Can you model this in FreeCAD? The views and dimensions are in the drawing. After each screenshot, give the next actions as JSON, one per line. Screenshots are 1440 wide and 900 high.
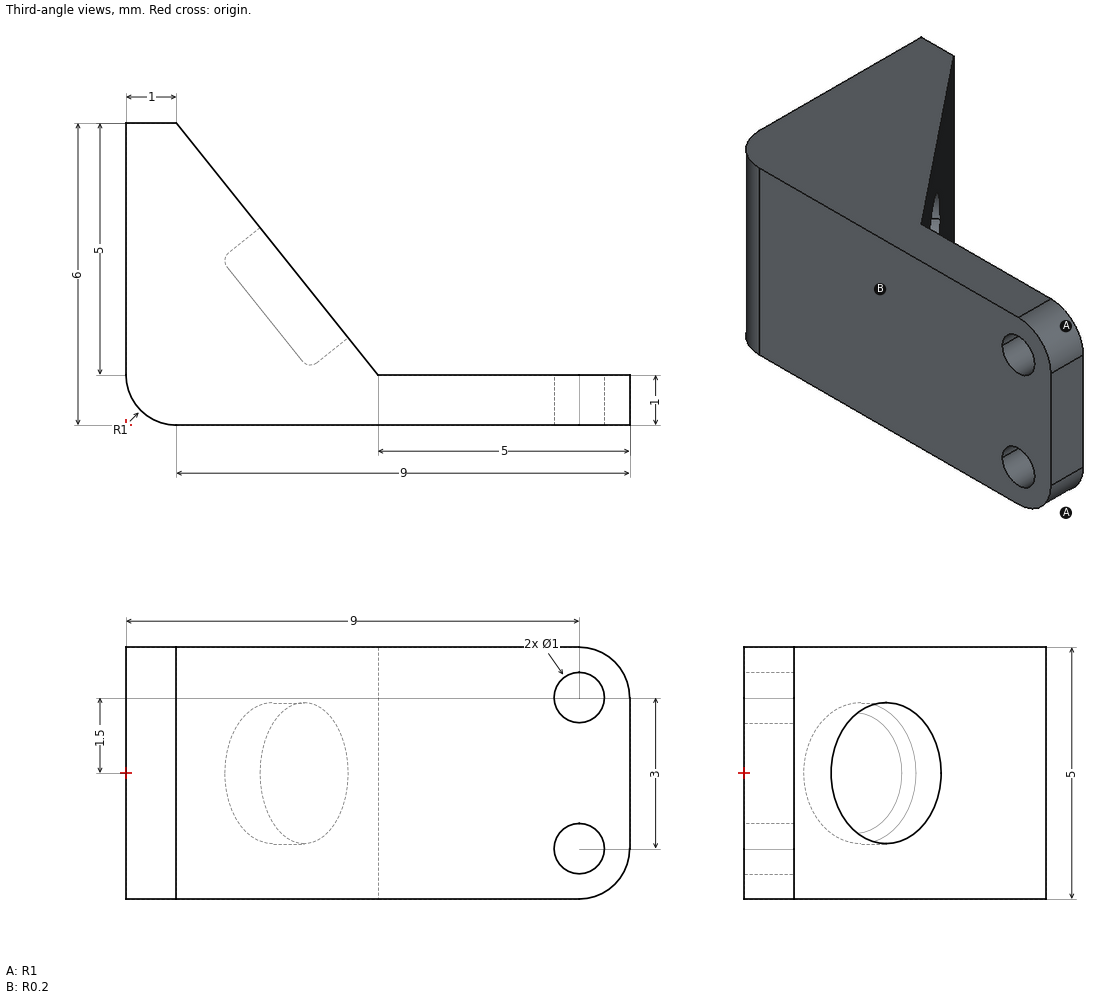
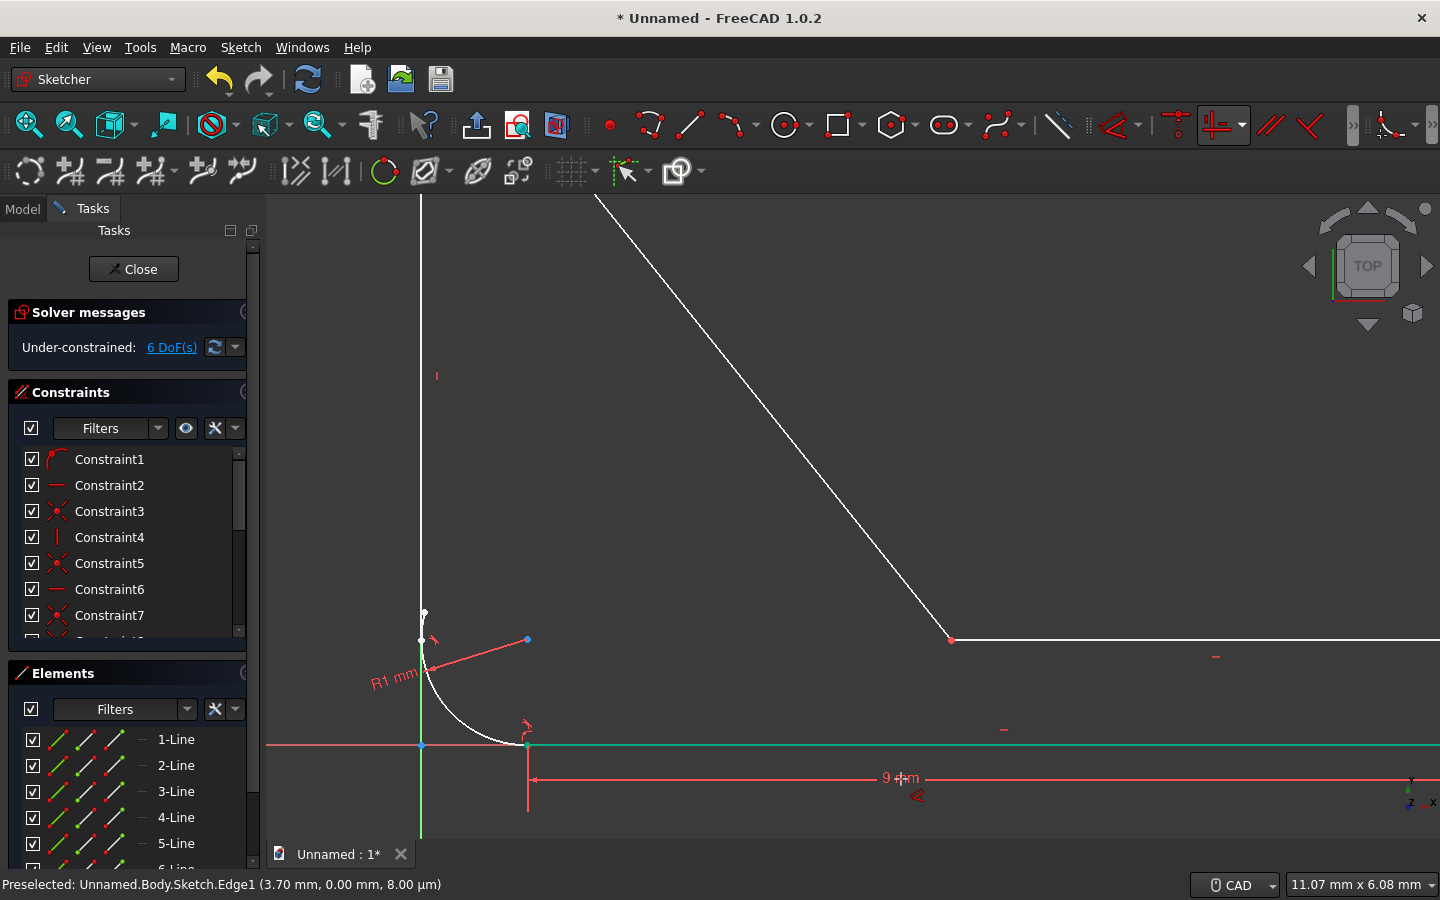
{"action": "scroll", "coordinate": [444, 698], "scroll_direction": "down", "scroll_amount": 2}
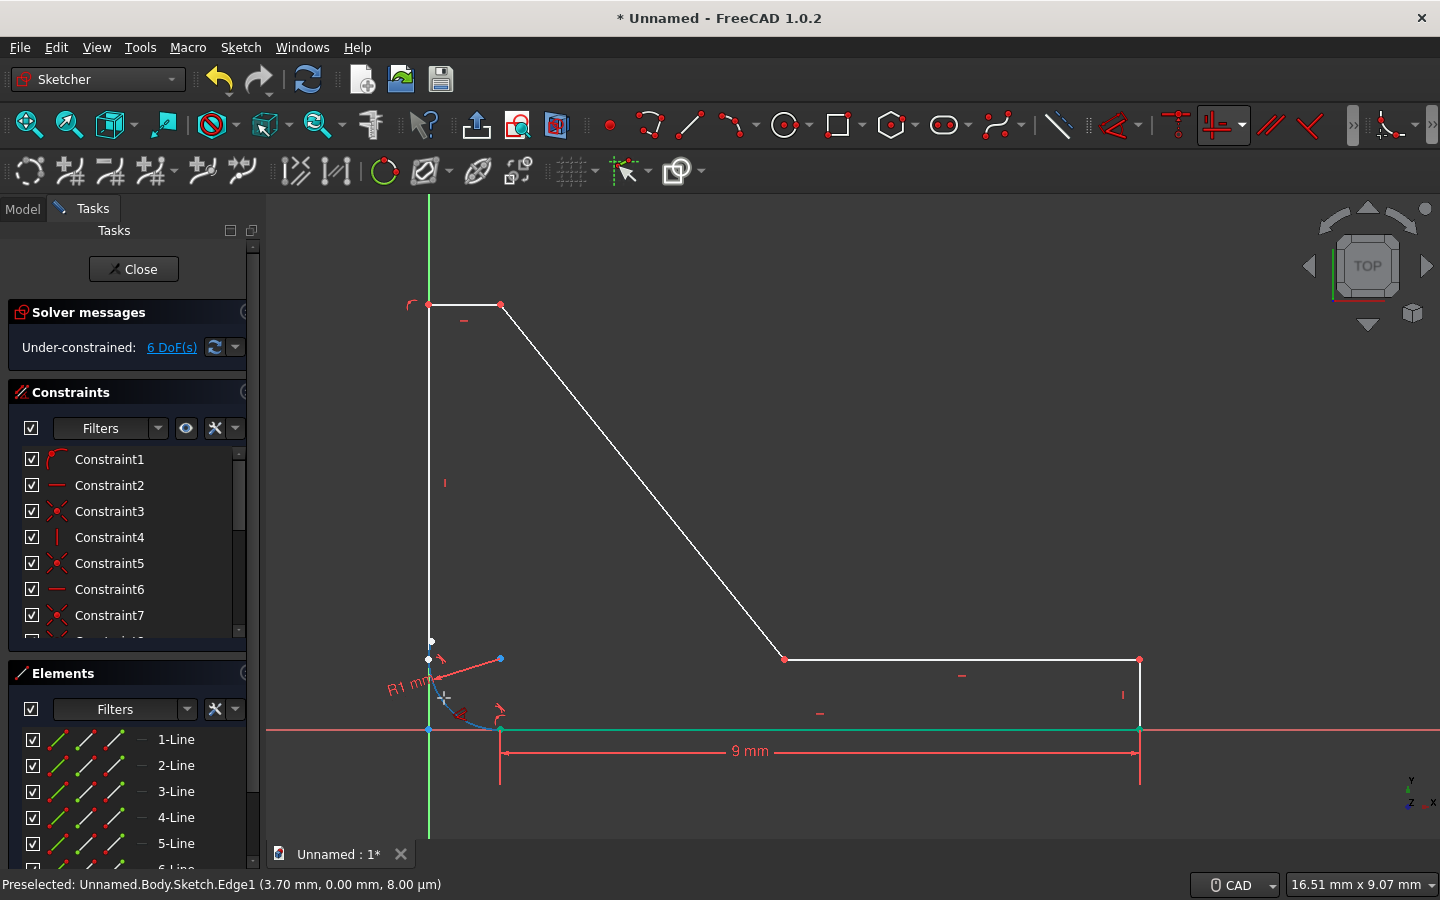
{"action": "left_click", "coordinate": [1140, 709]}
{"action": "left_click", "coordinate": [1174, 695]}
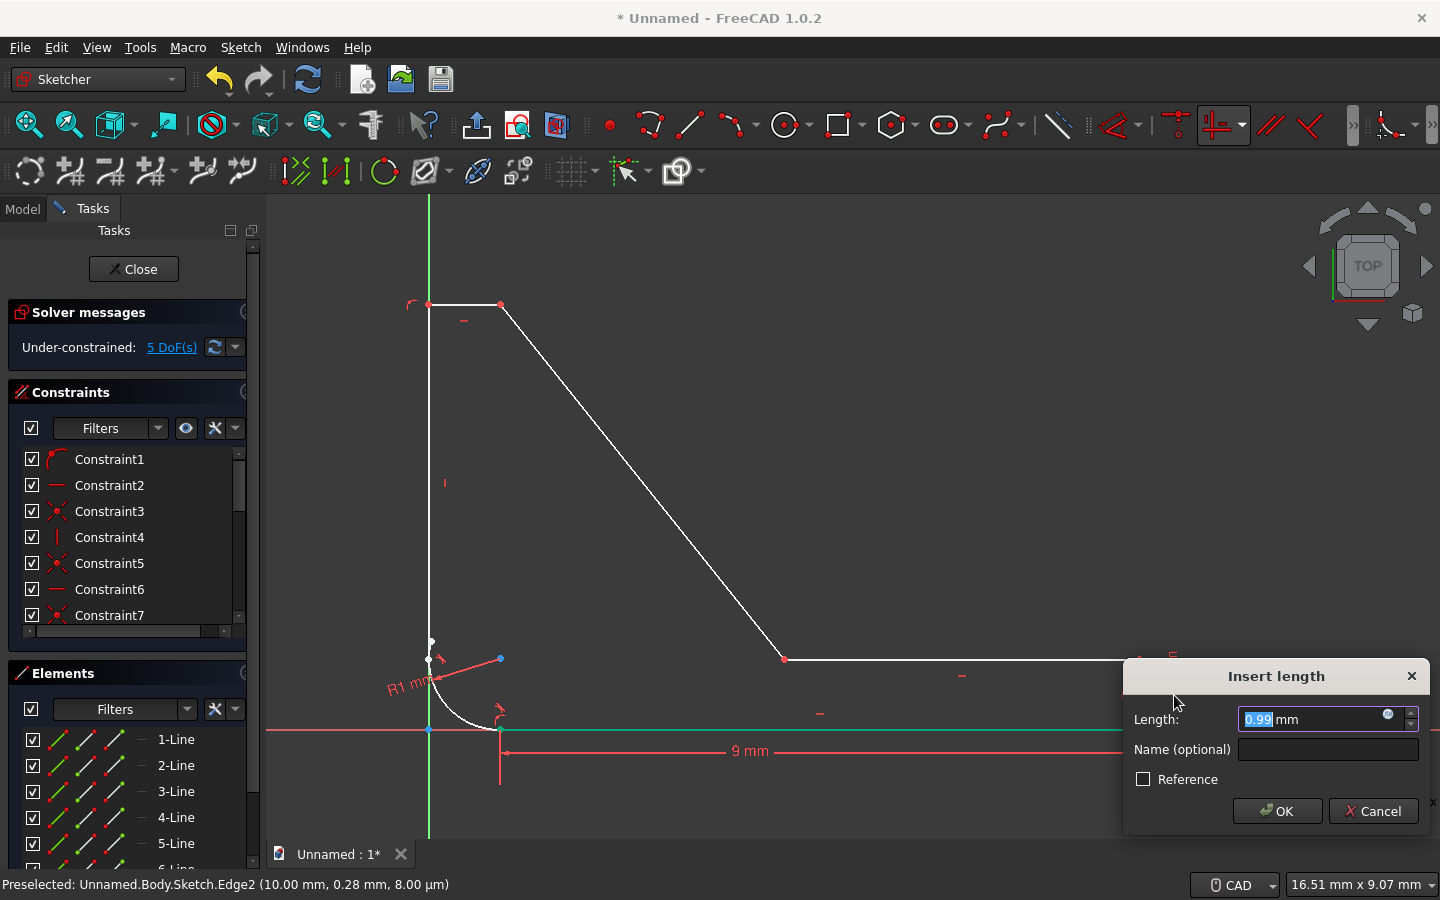
{"action": "type", "text": "1"}
{"action": "key", "text": "Return"}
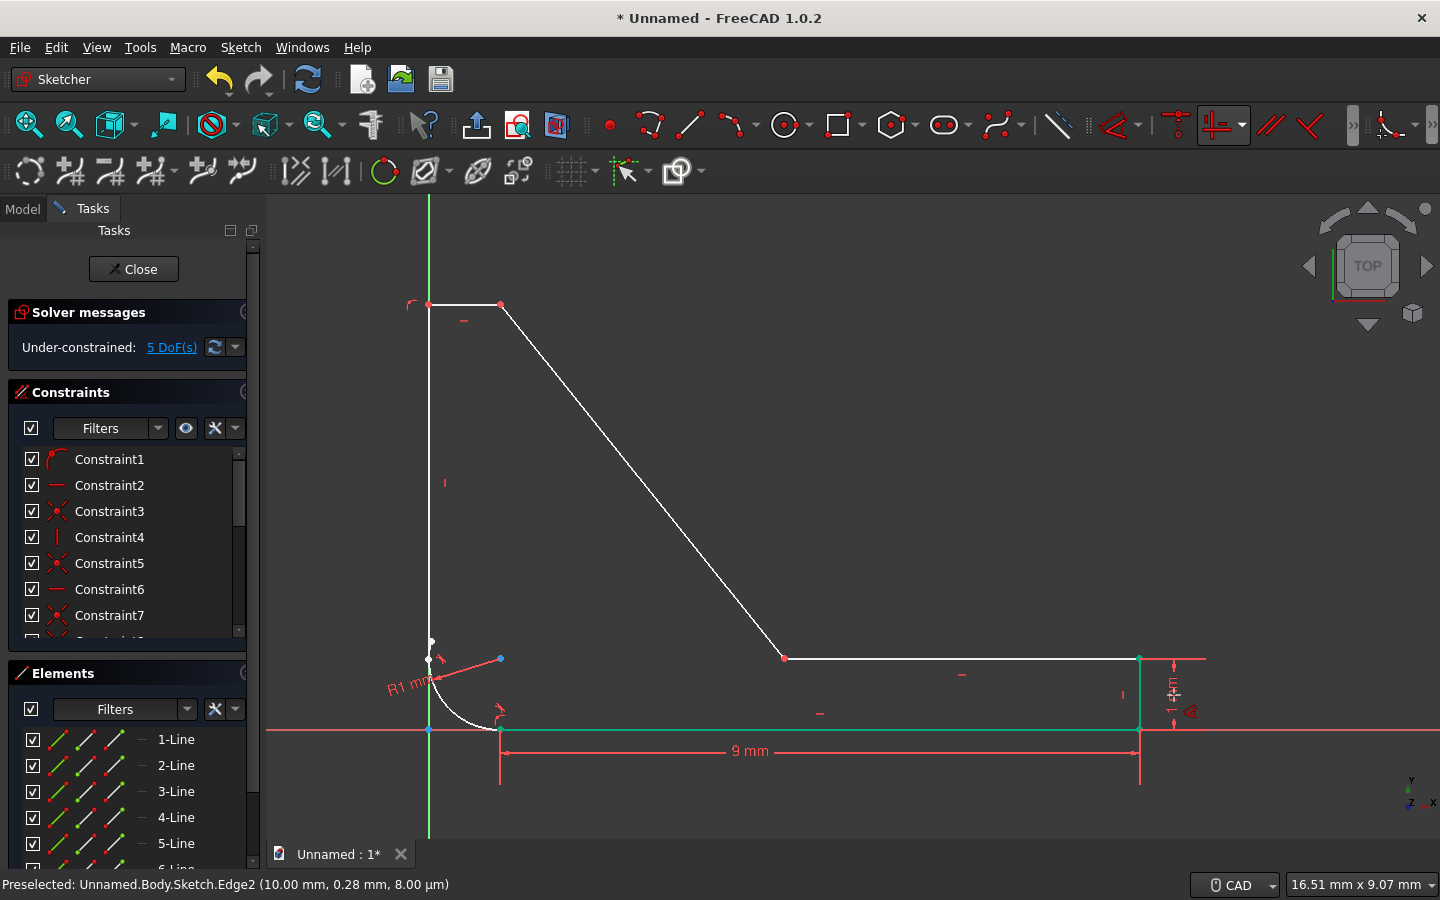
{"action": "left_click", "coordinate": [1033, 659]}
{"action": "left_click", "coordinate": [962, 693]}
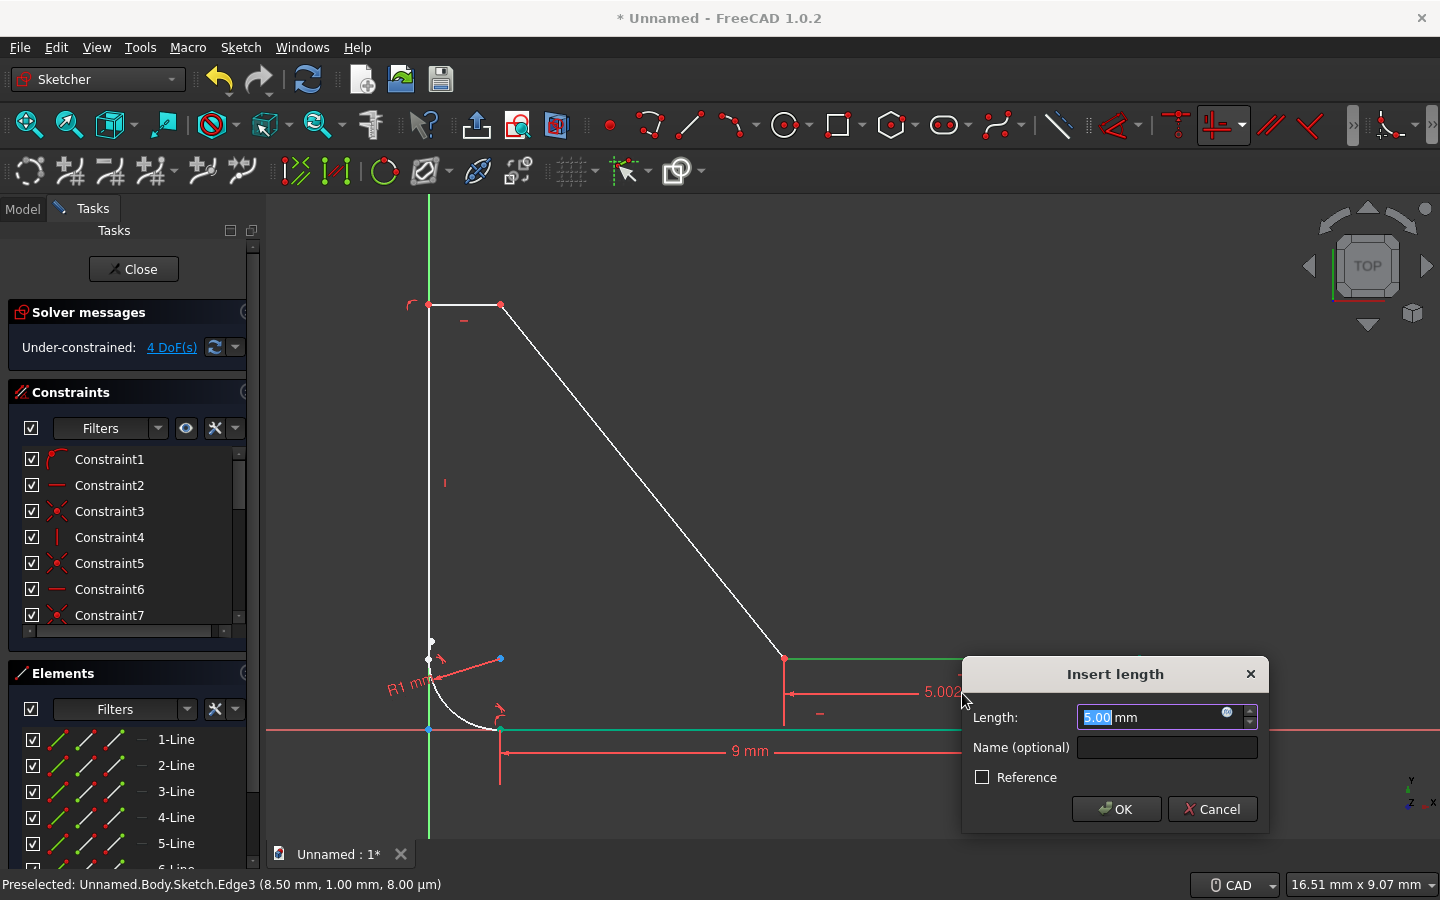
{"action": "type", "text": "5"}
{"action": "key", "text": "Return"}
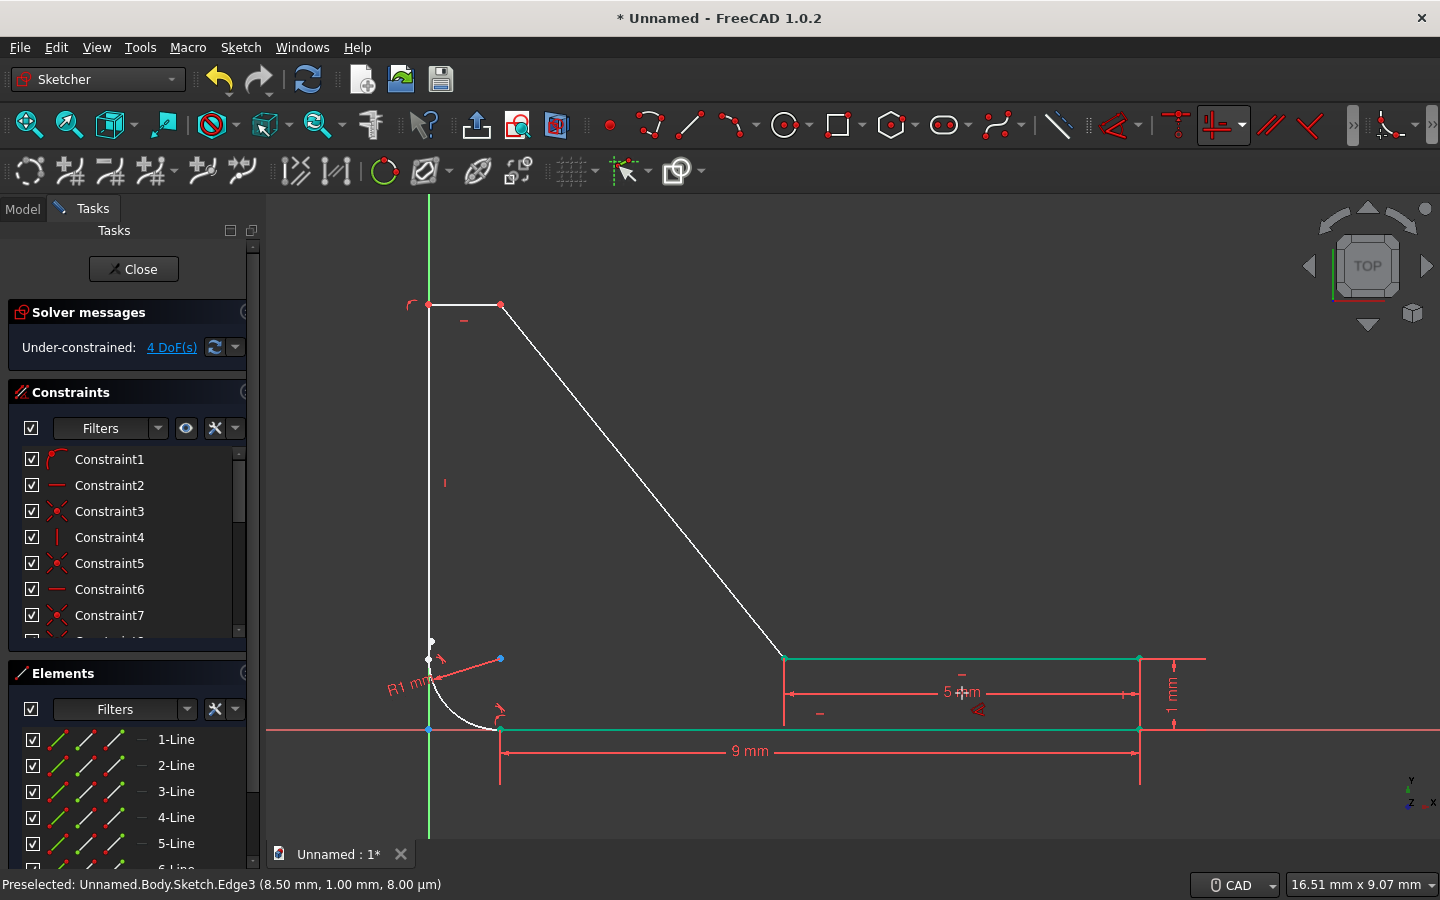
{"action": "left_click", "coordinate": [479, 305]}
{"action": "left_click", "coordinate": [465, 271]}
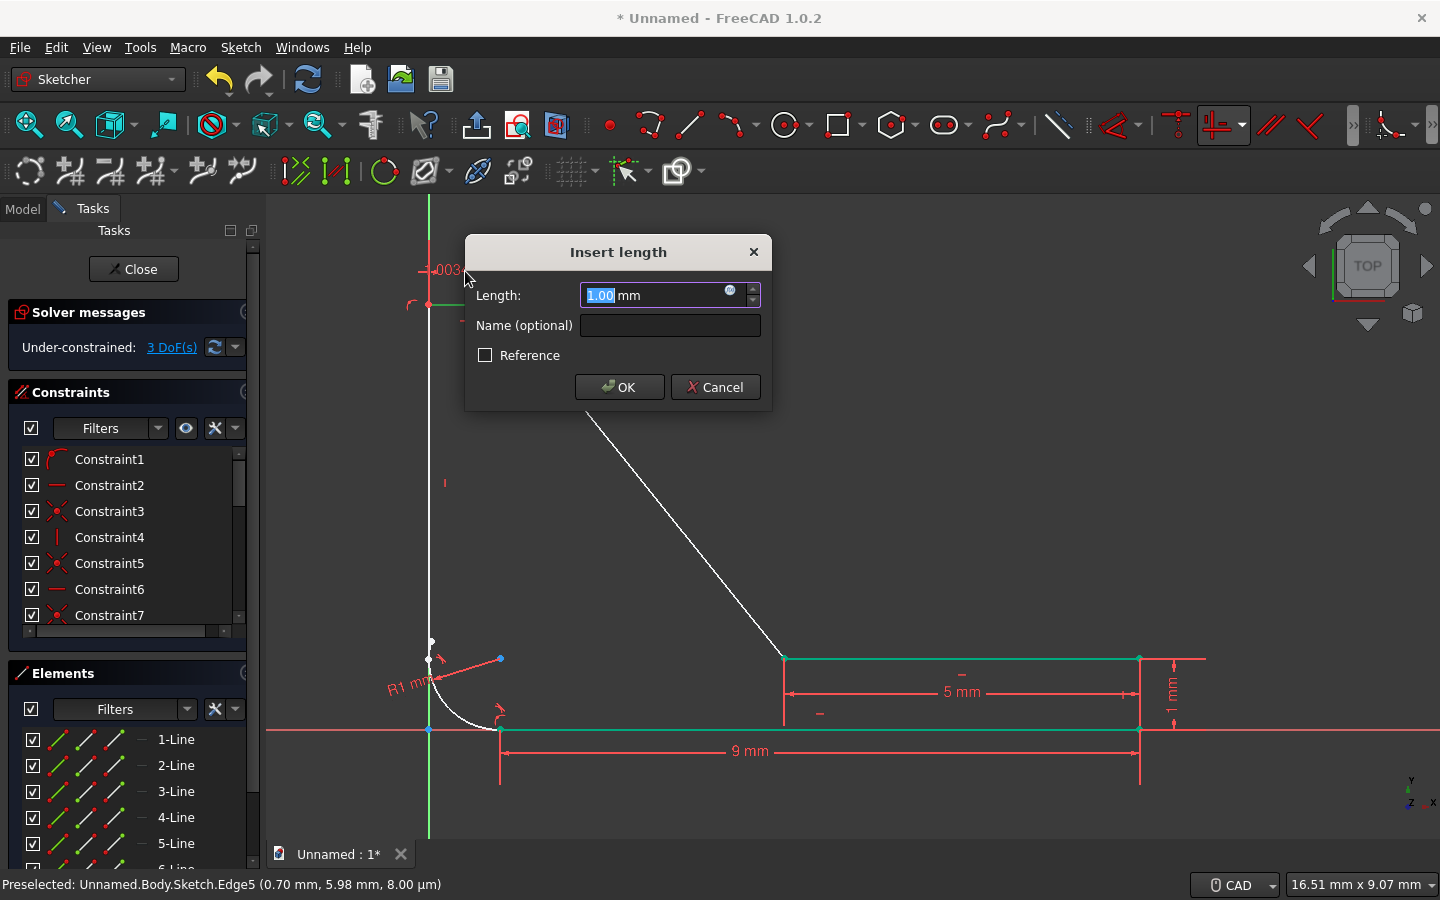
{"action": "type", "text": "1"}
{"action": "key", "text": "Return"}